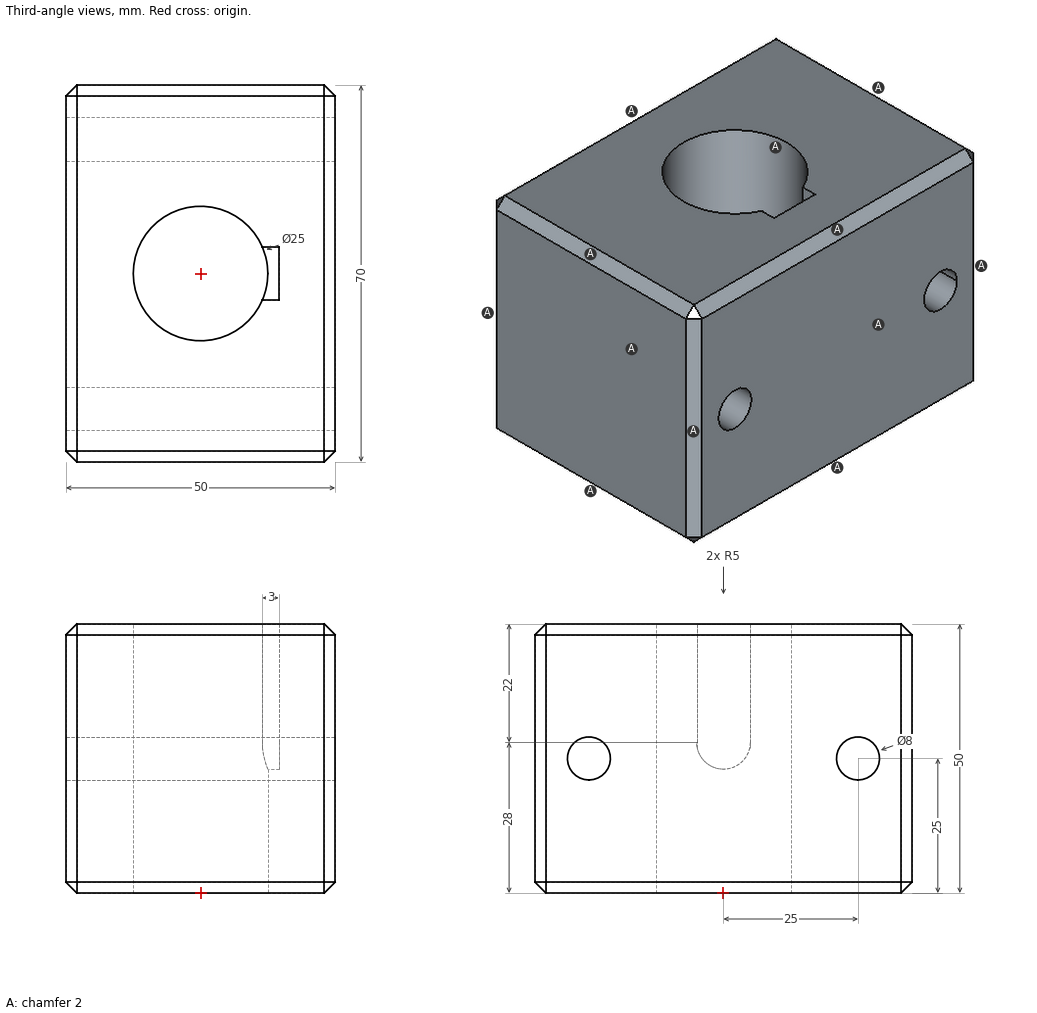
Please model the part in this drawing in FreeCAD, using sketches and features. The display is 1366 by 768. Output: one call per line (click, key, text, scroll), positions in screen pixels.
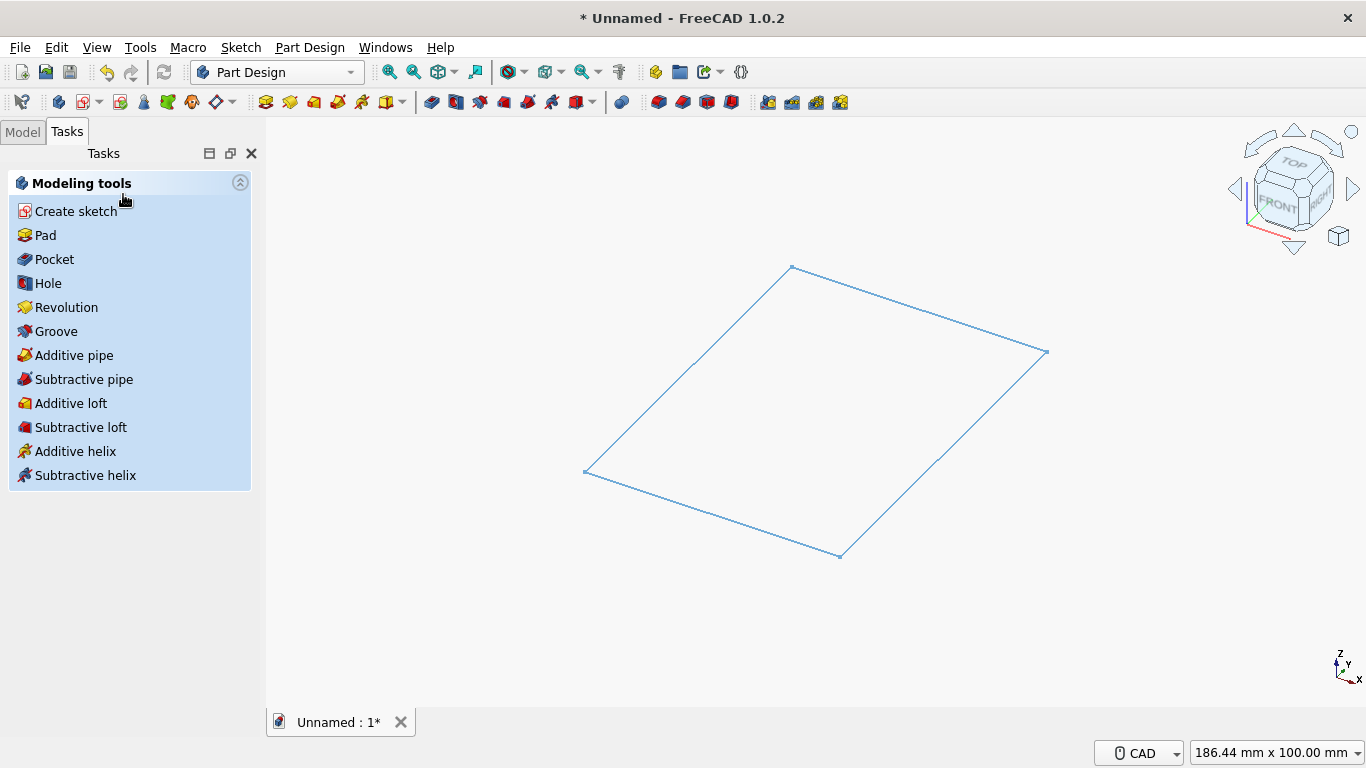
click(266, 102)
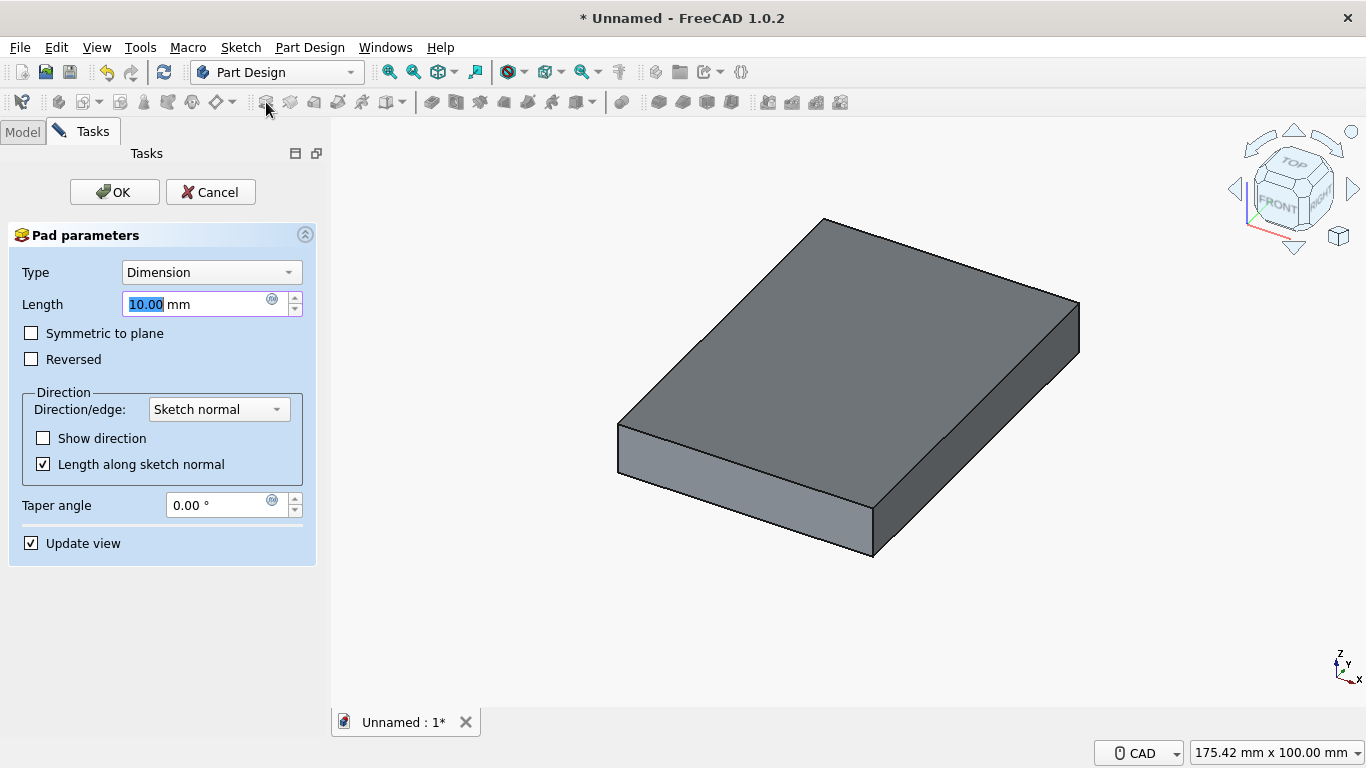
text(50)
key(Tab)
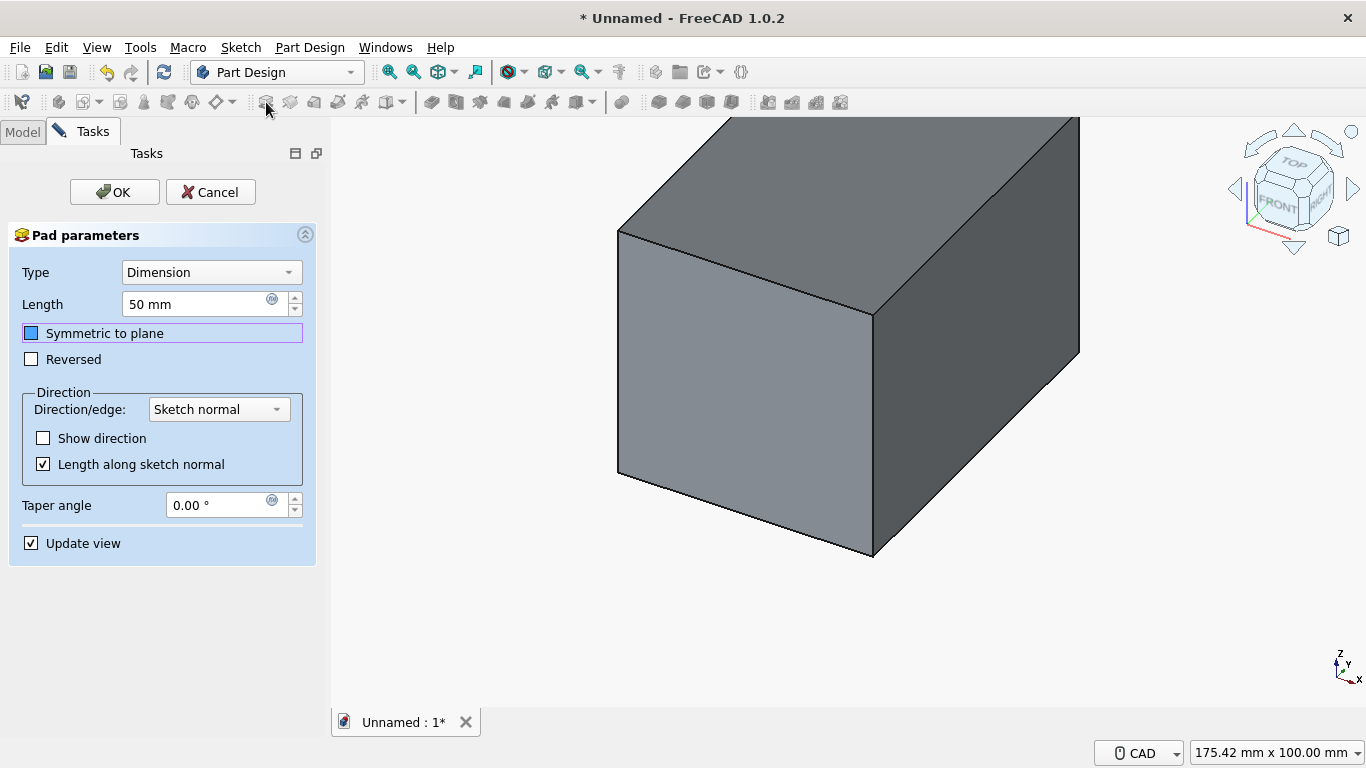
click(115, 192)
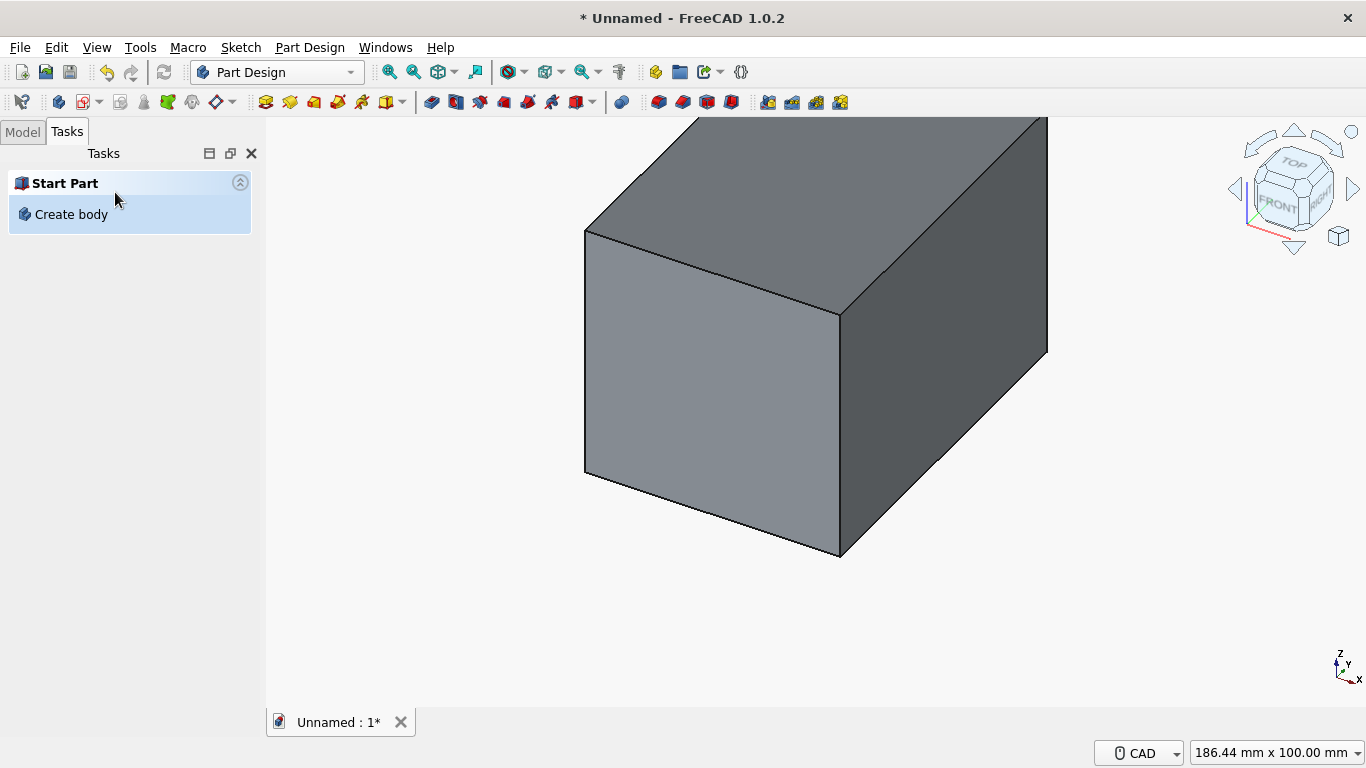
click(390, 72)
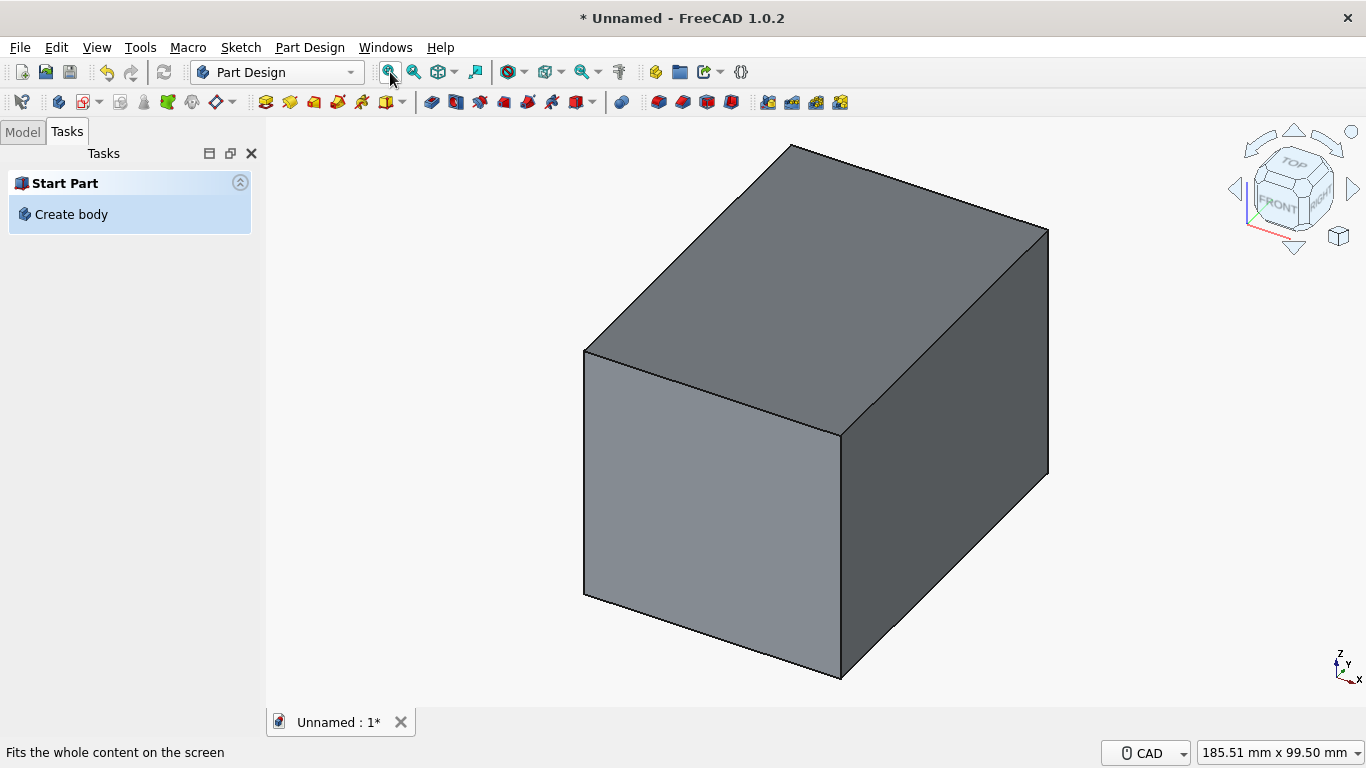
click(846, 260)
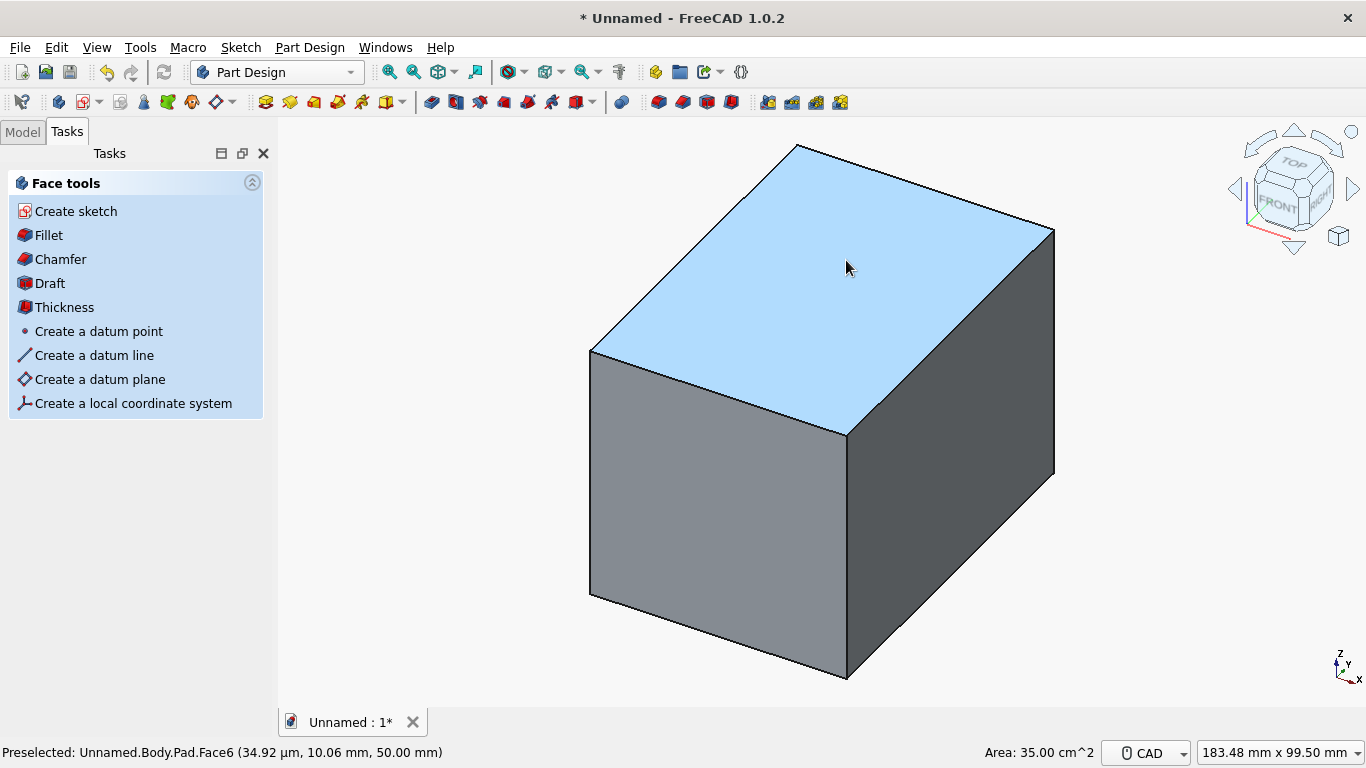
click(84, 102)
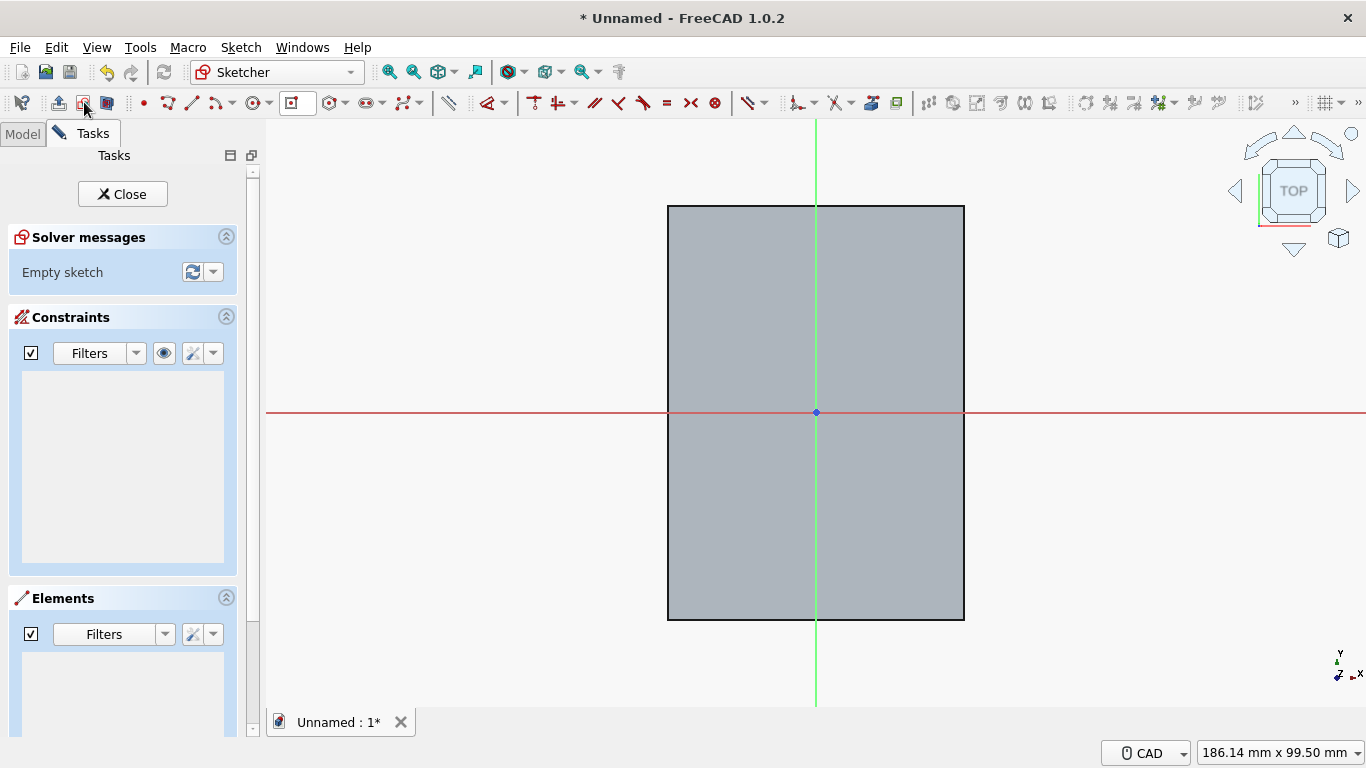
scroll(856, 413, up, 5)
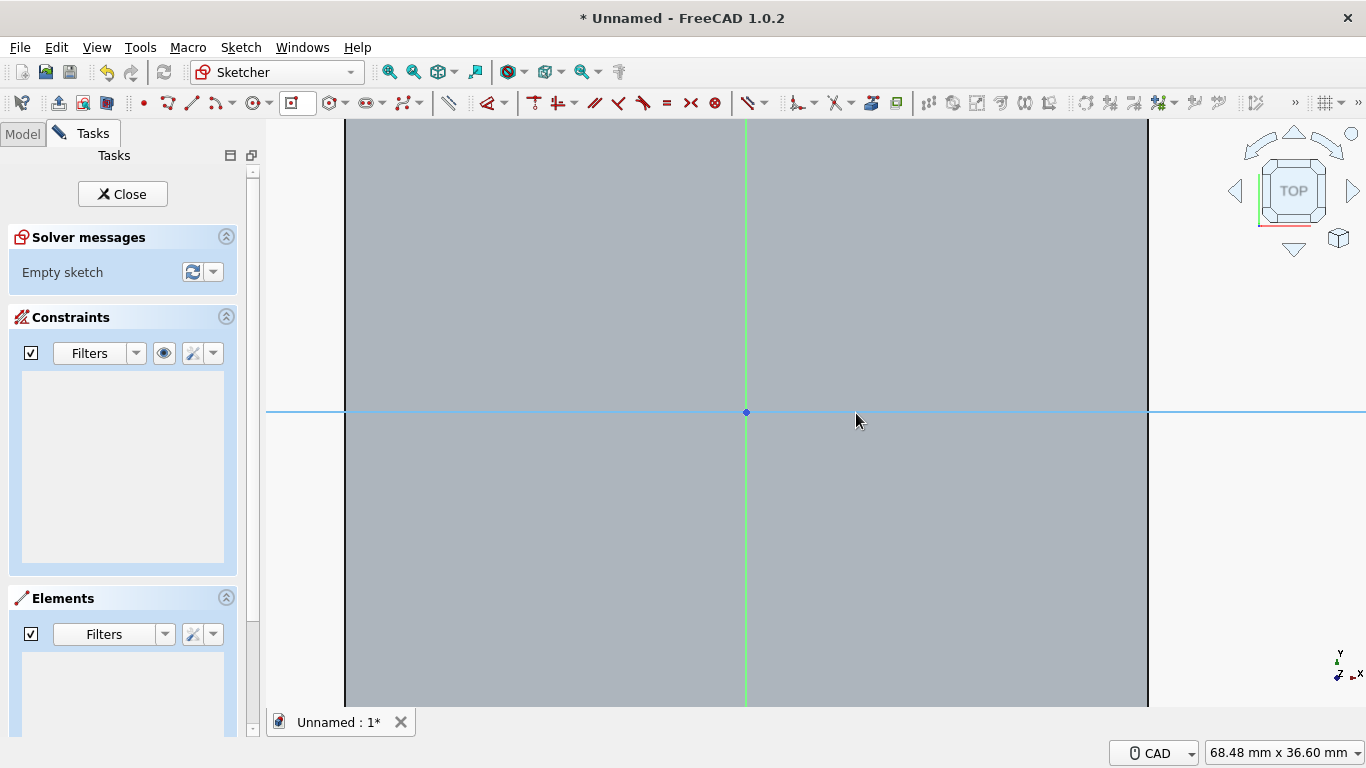
click(254, 104)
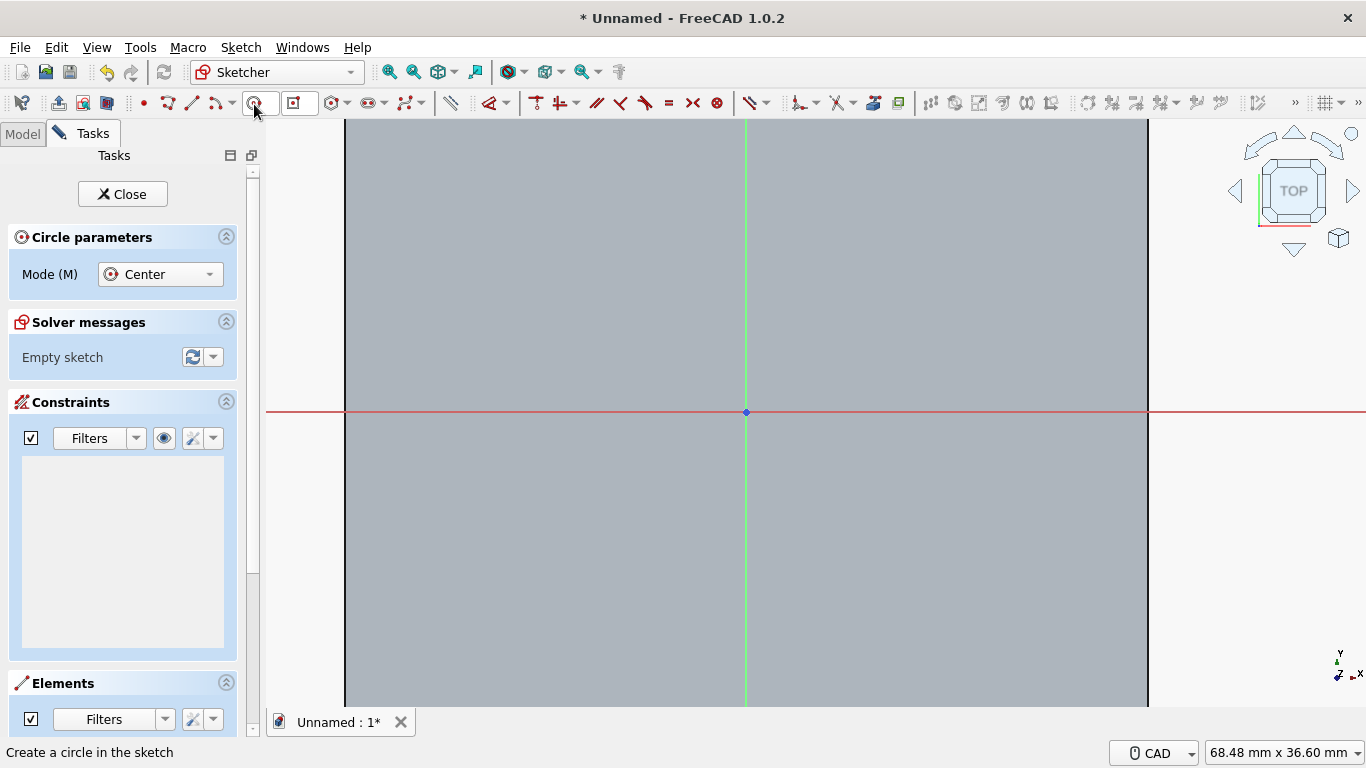
click(746, 412)
move(888, 270)